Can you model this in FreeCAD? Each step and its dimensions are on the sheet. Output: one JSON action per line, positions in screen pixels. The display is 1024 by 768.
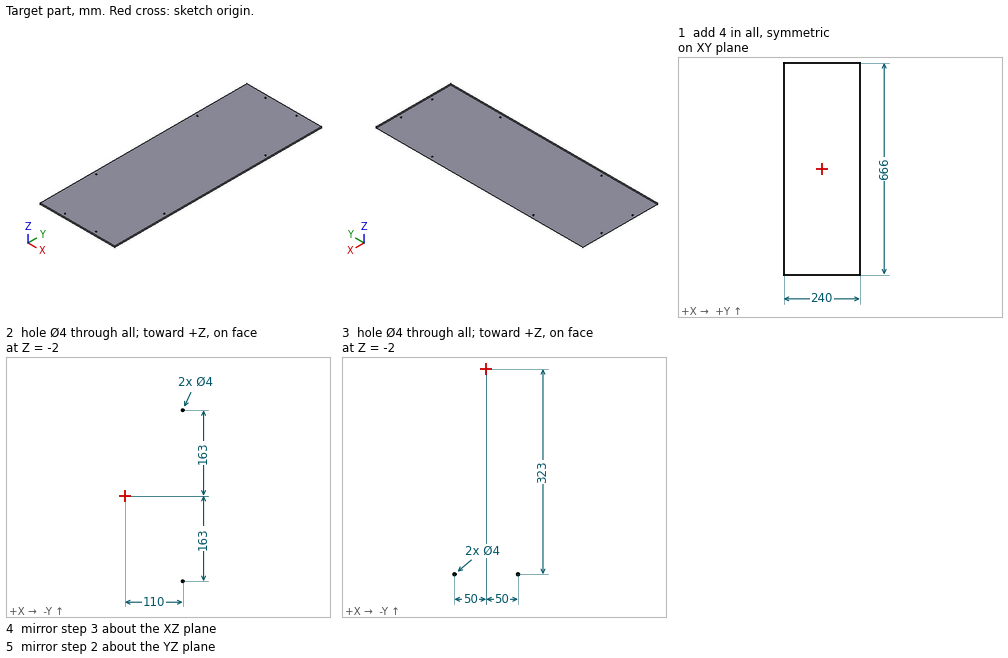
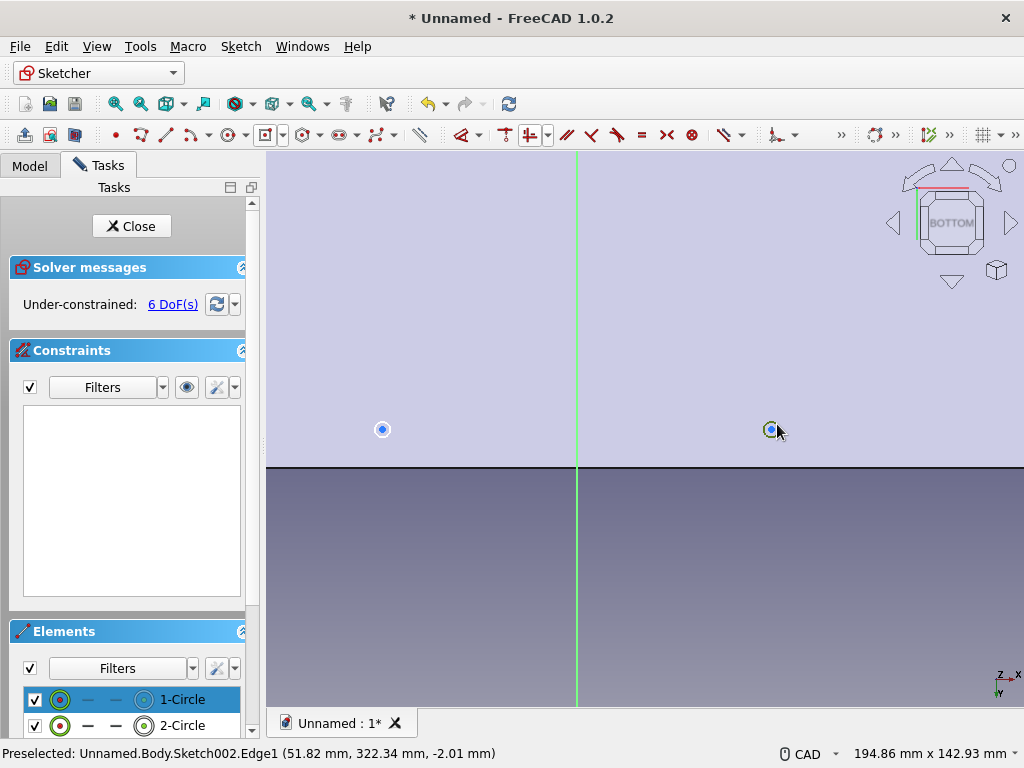
{"action": "scroll", "coordinate": [388, 424], "scroll_direction": "up", "scroll_amount": 3}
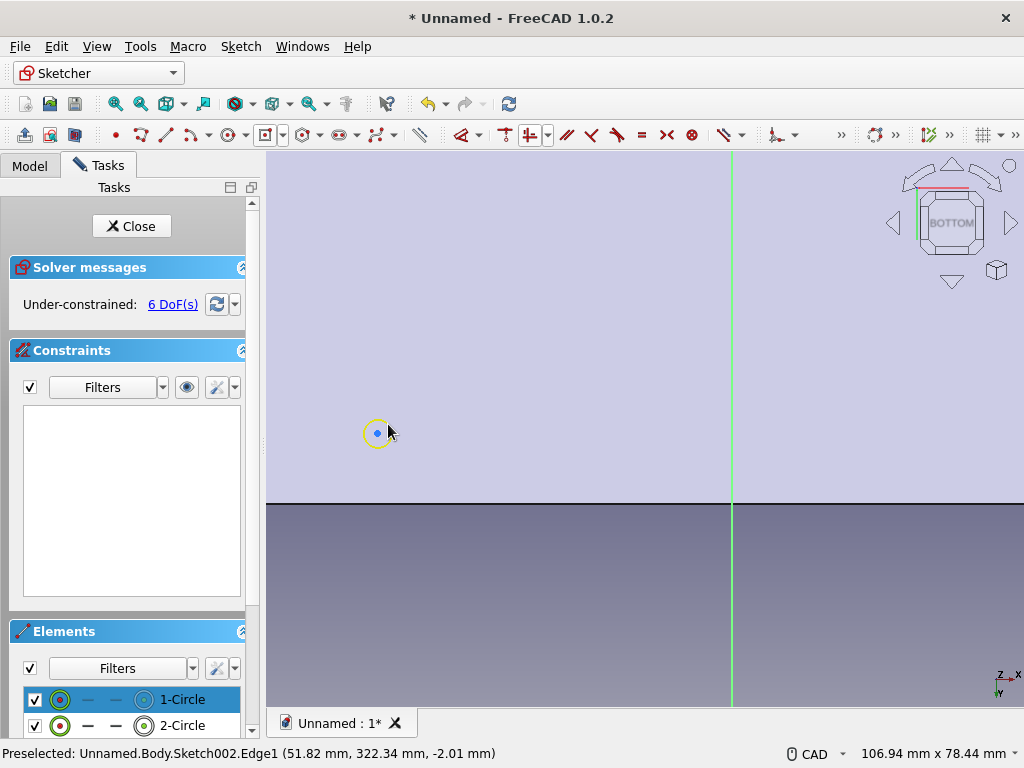
{"action": "left_click", "coordinate": [388, 424]}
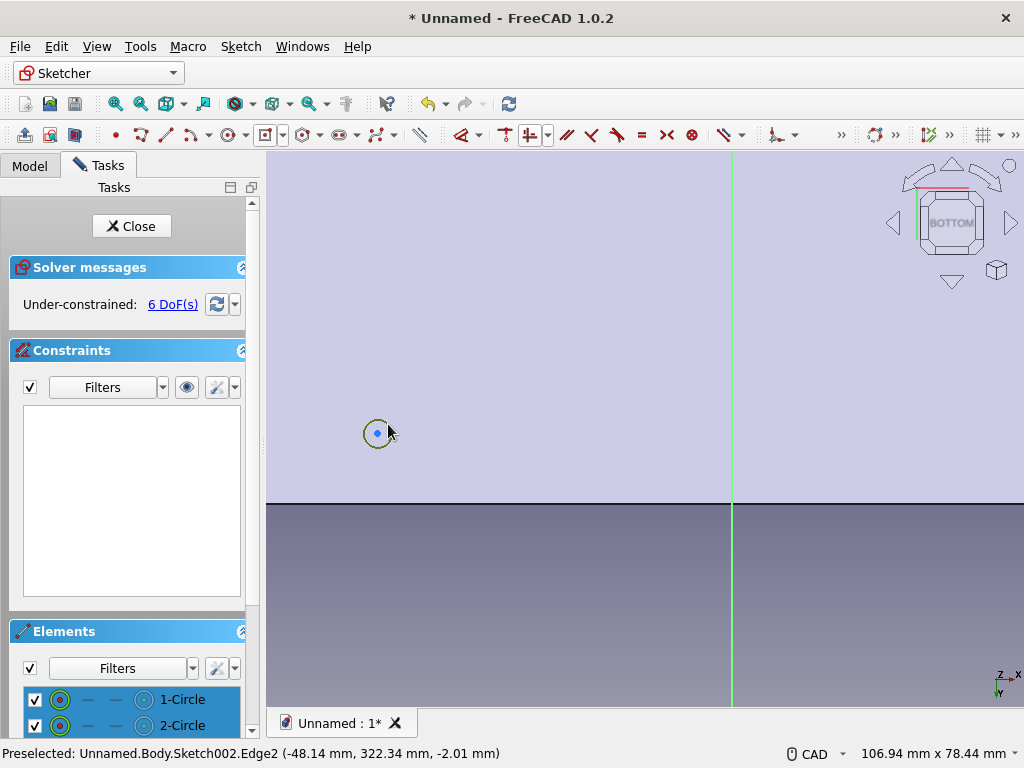
{"action": "left_click", "coordinate": [642, 136]}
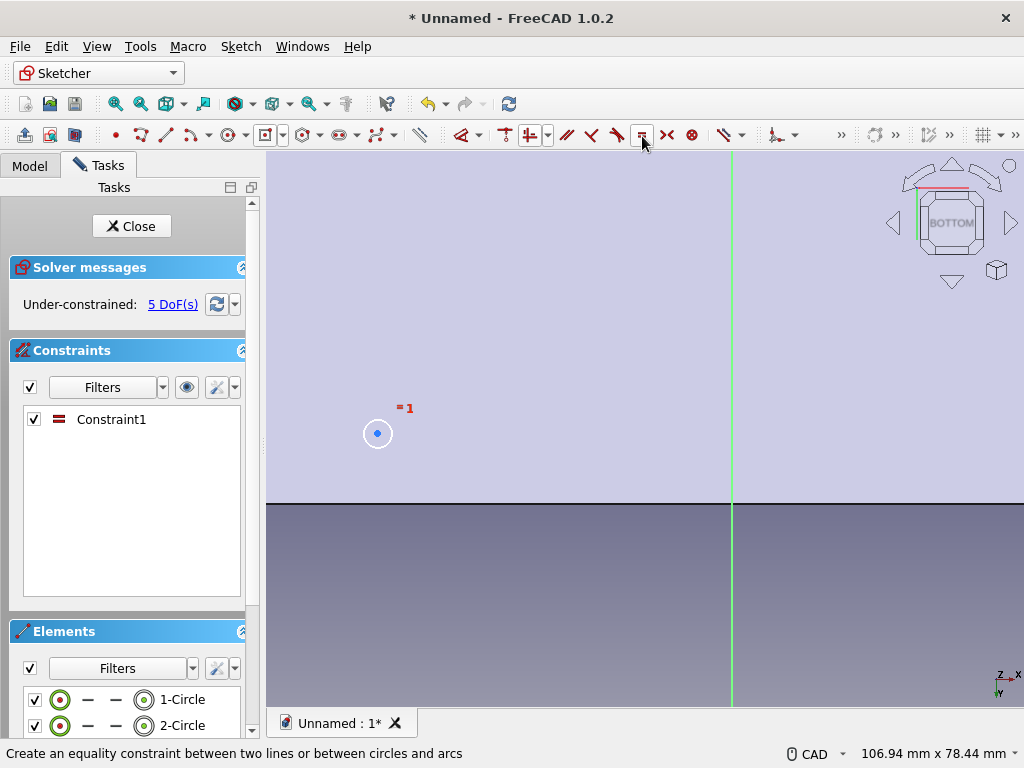
{"action": "scroll", "coordinate": [387, 424], "scroll_direction": "down", "scroll_amount": 3}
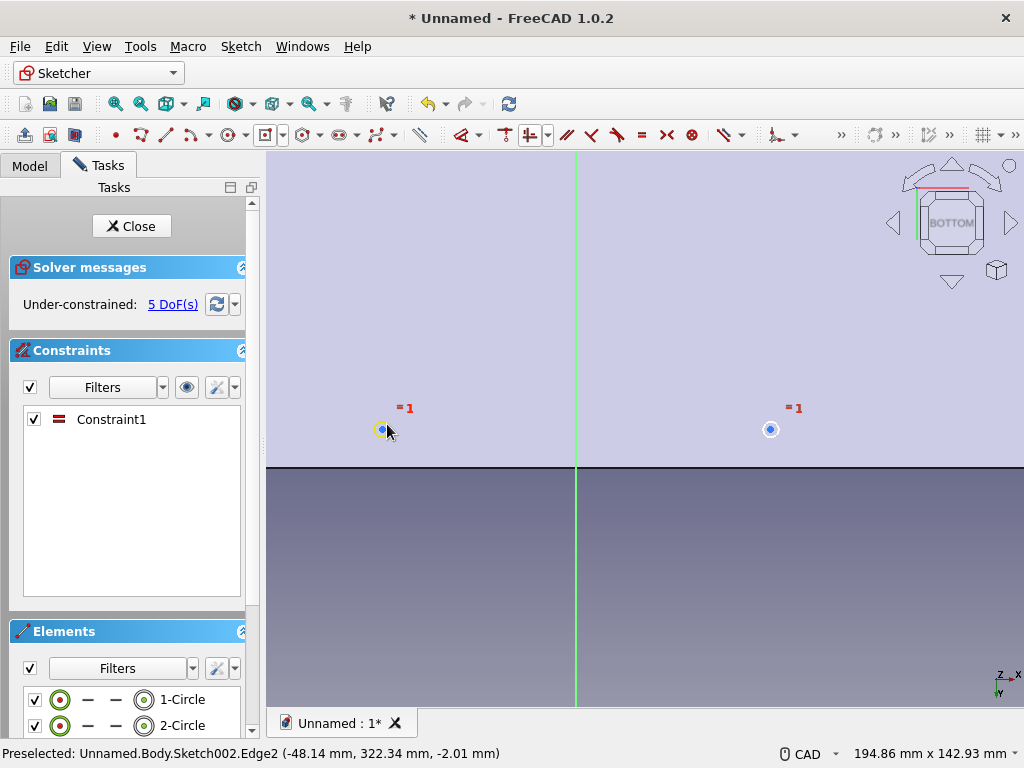
{"action": "left_click", "coordinate": [771, 430]}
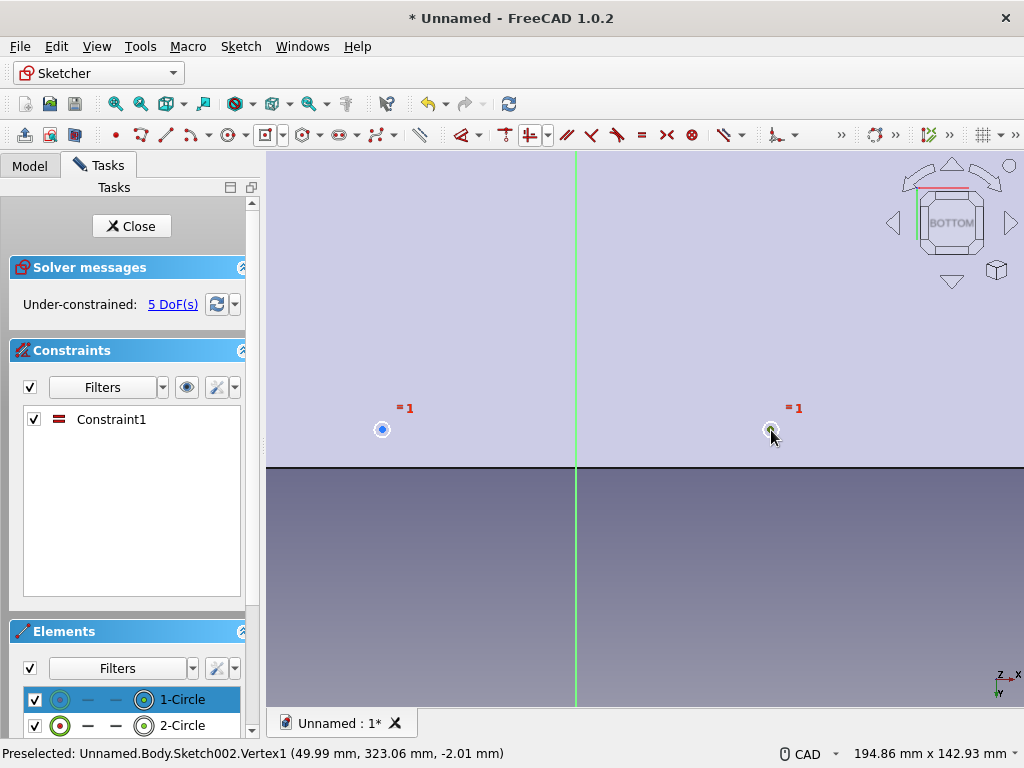
{"action": "left_click", "coordinate": [382, 430]}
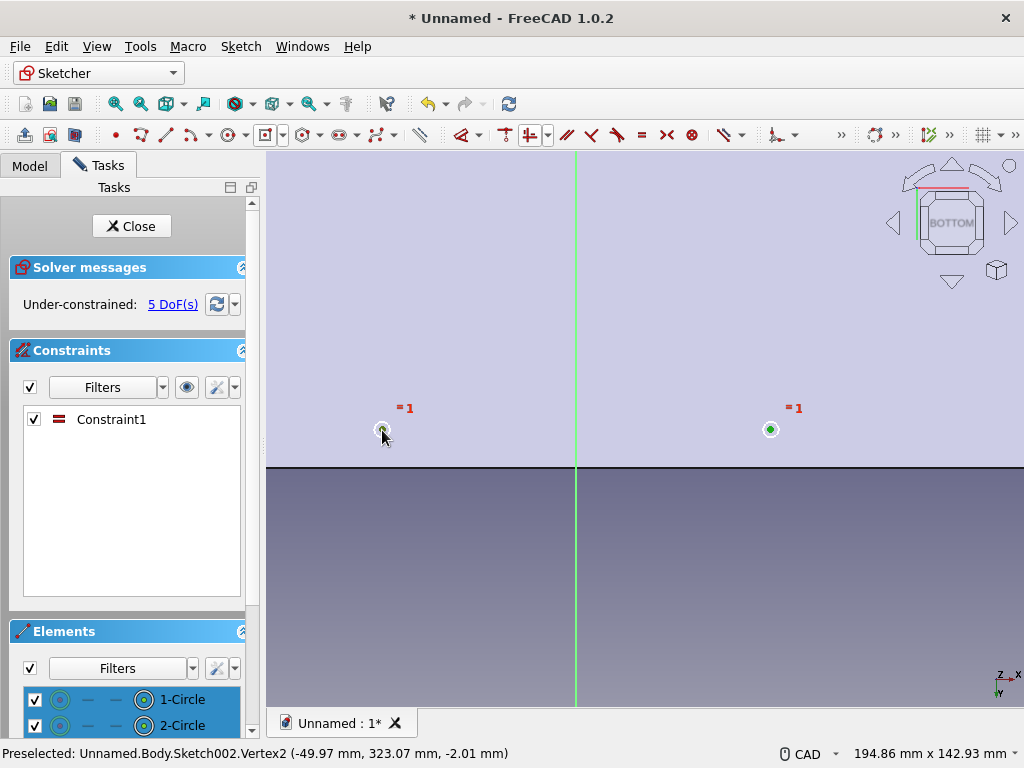
{"action": "key", "text": "h"}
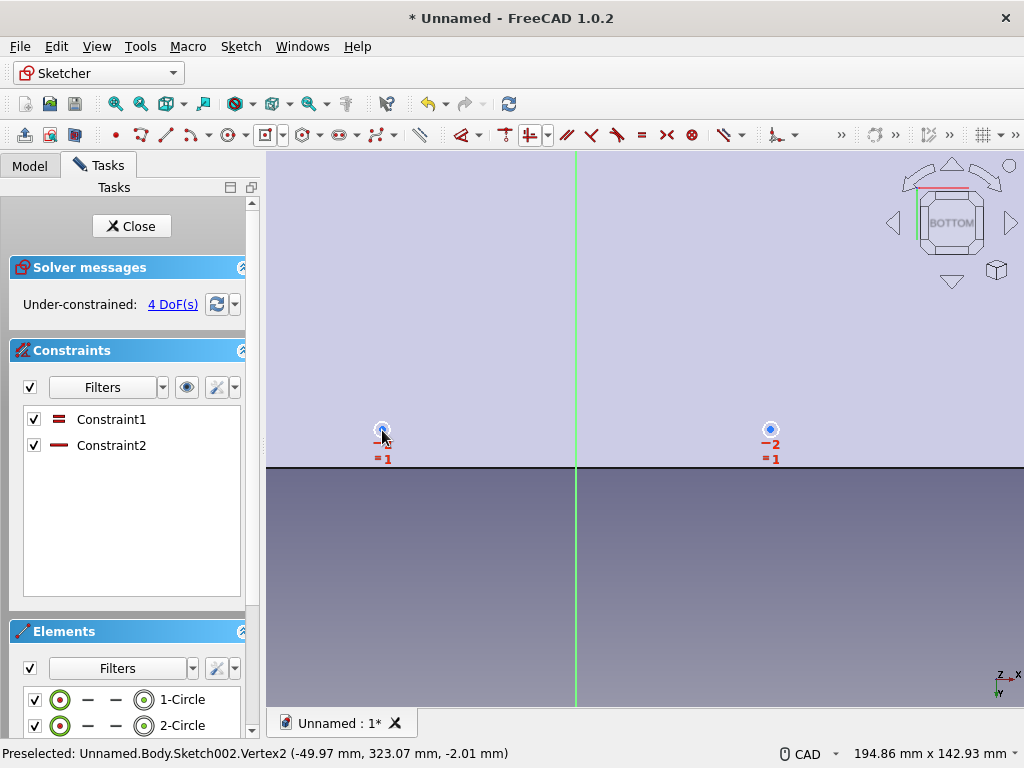
{"action": "left_click", "coordinate": [460, 136]}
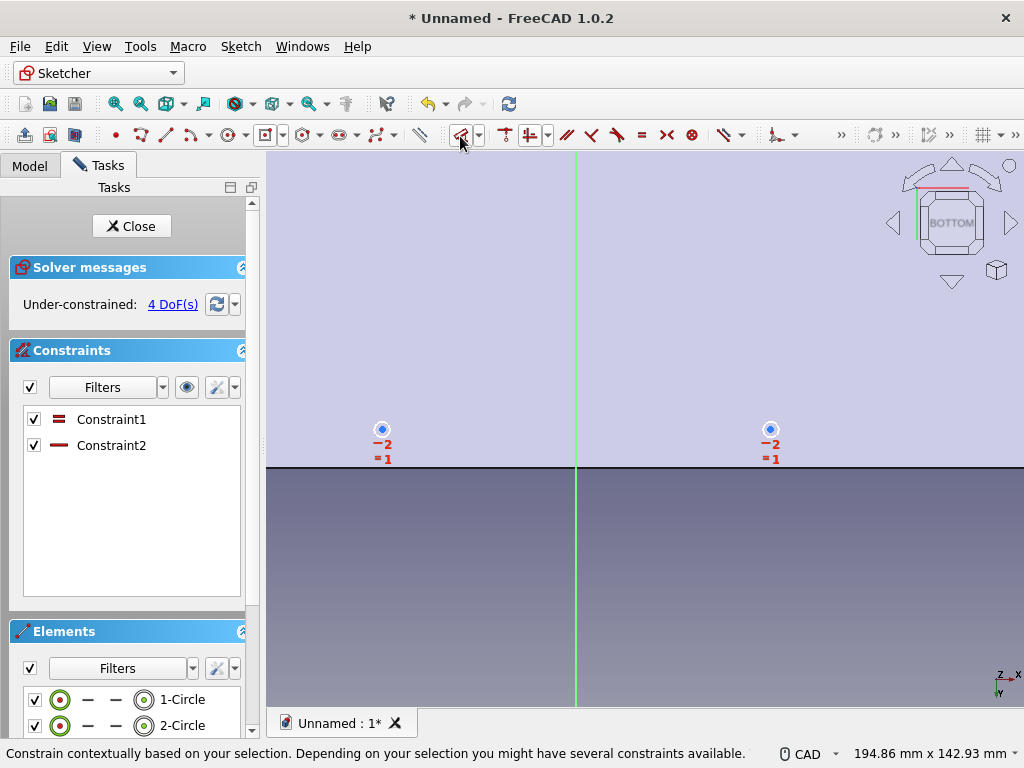
{"action": "scroll", "coordinate": [776, 424], "scroll_direction": "up", "scroll_amount": 5}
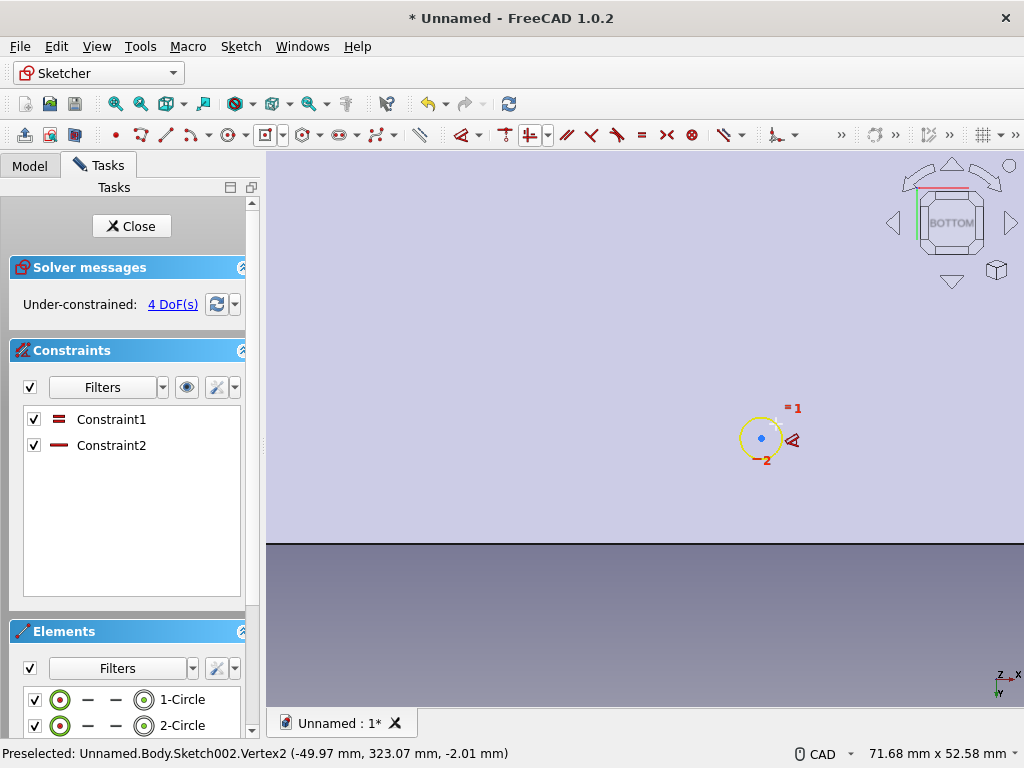
{"action": "left_click", "coordinate": [776, 424]}
{"action": "left_click", "coordinate": [799, 402]}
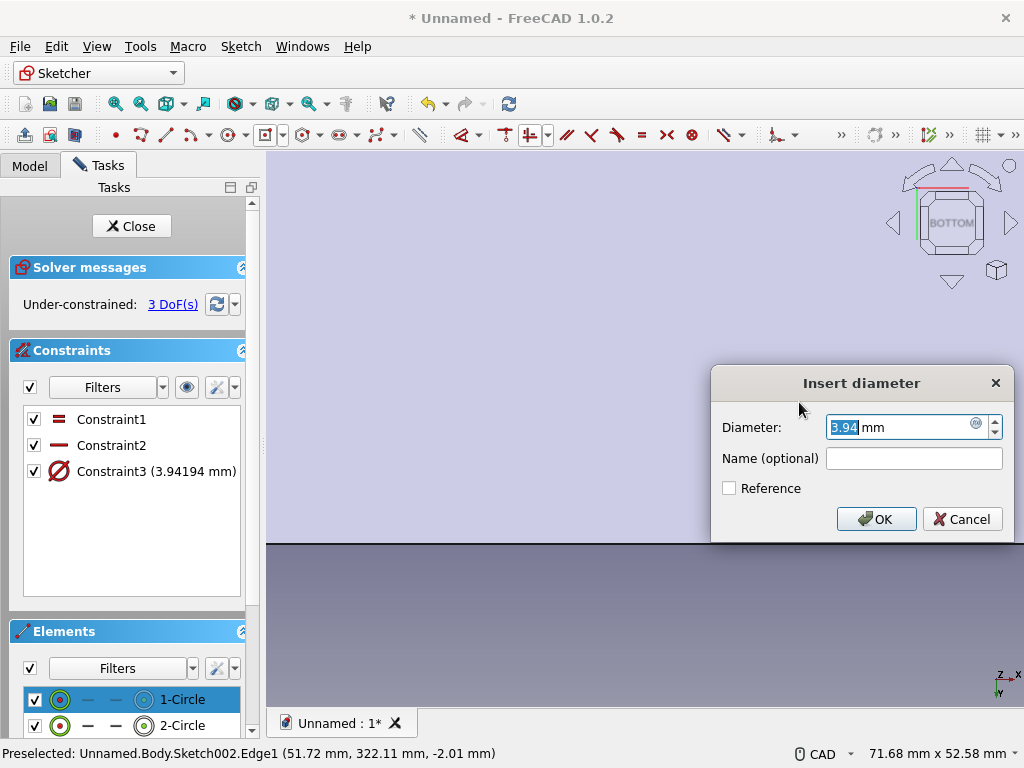
{"action": "type", "text": "4"}
{"action": "key", "text": "Return"}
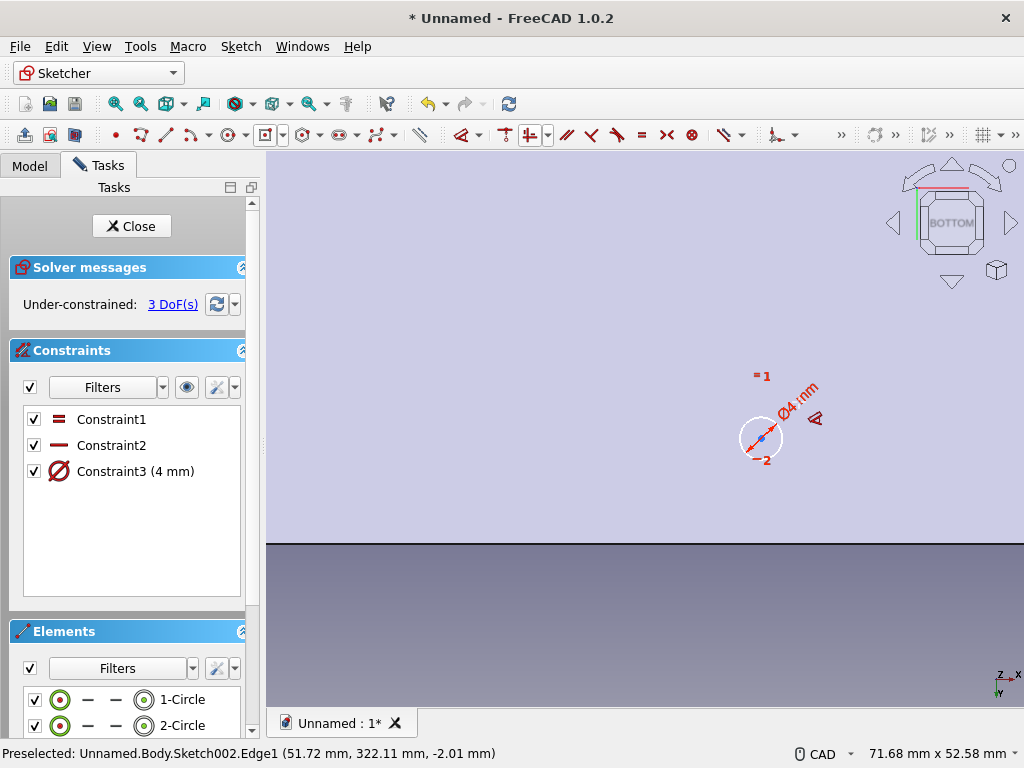
{"action": "left_click", "coordinate": [761, 438]}
{"action": "left_click", "coordinate": [528, 472]}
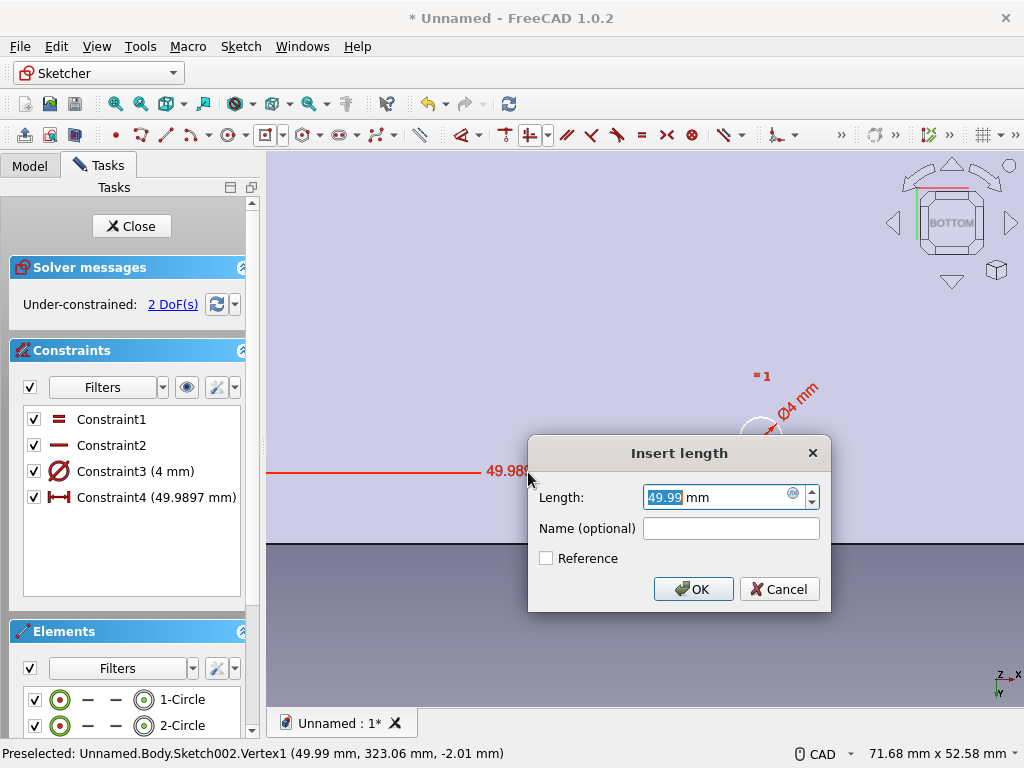
{"action": "type", "text": "50"}
{"action": "key", "text": "Return"}